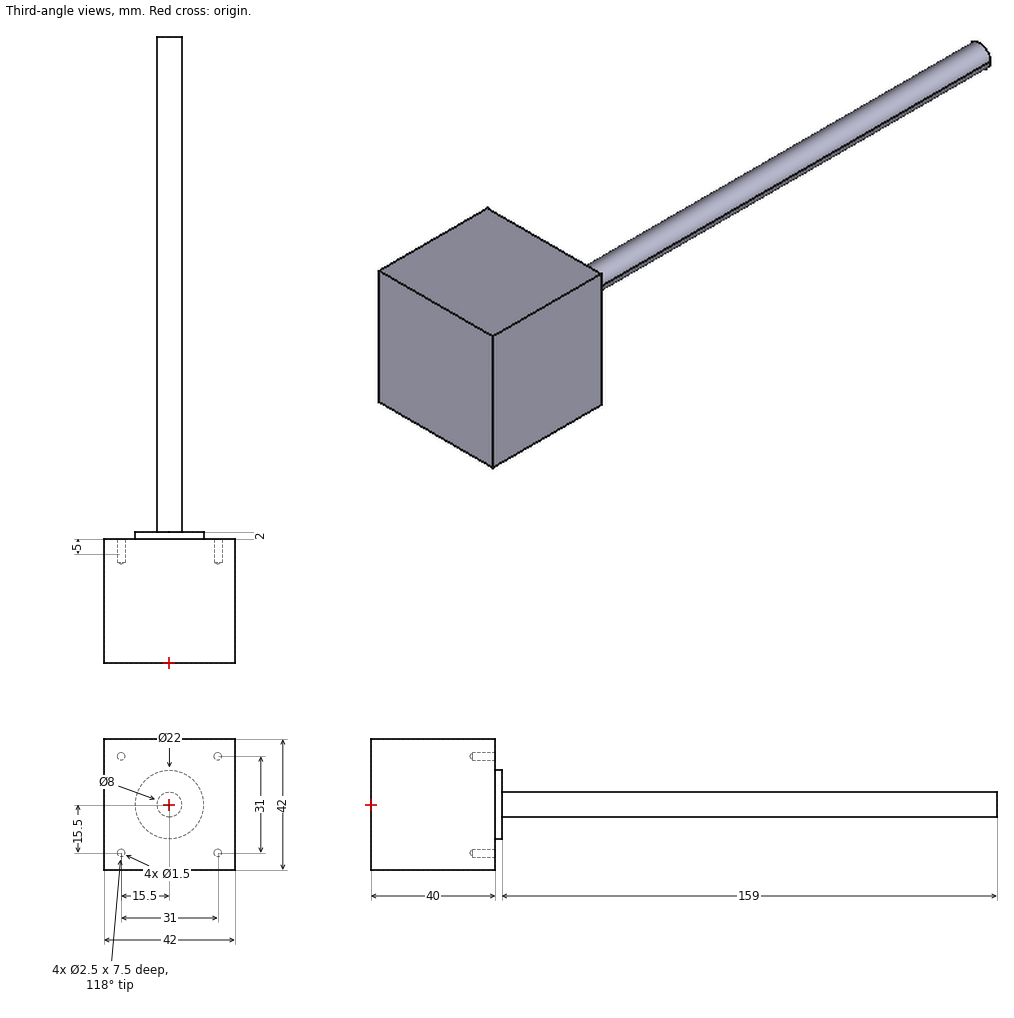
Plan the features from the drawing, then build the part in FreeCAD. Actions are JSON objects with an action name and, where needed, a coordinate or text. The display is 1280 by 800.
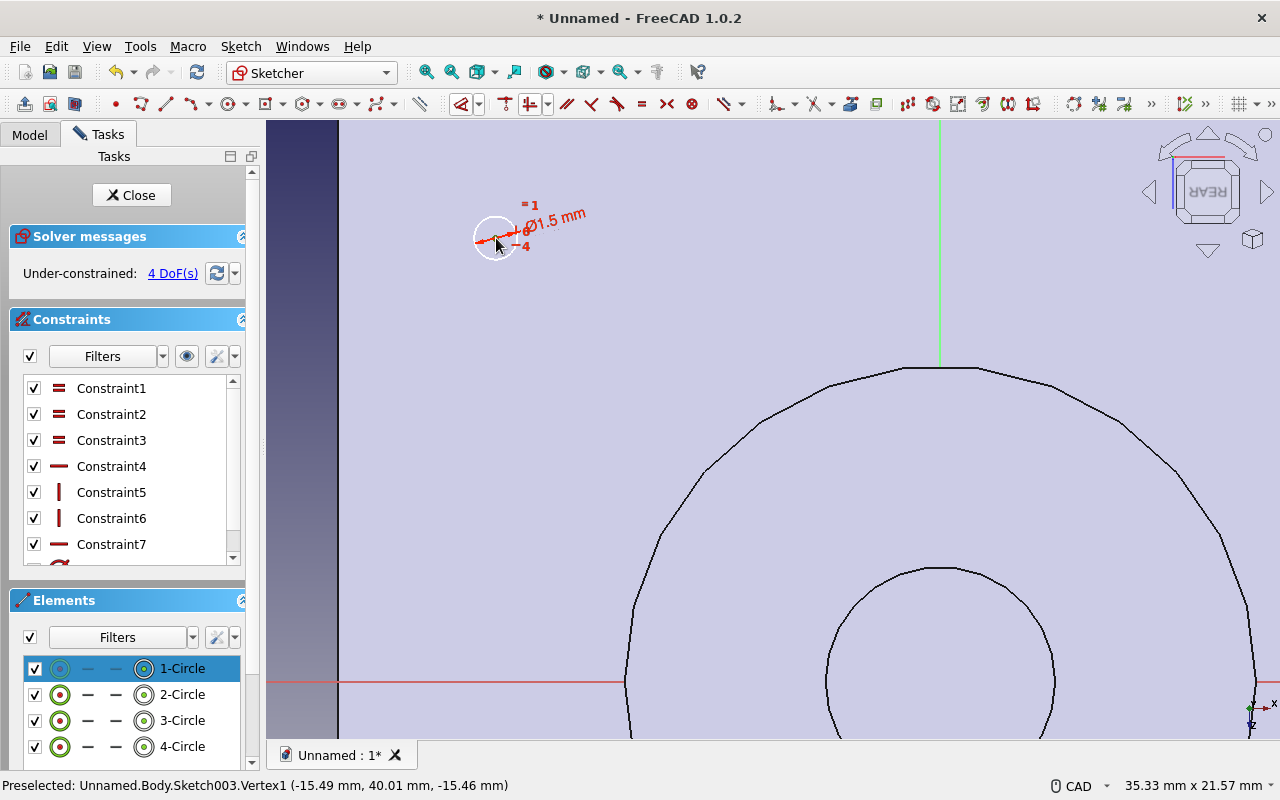
{"action": "scroll", "coordinate": [512, 224], "scroll_direction": "down", "scroll_amount": 4}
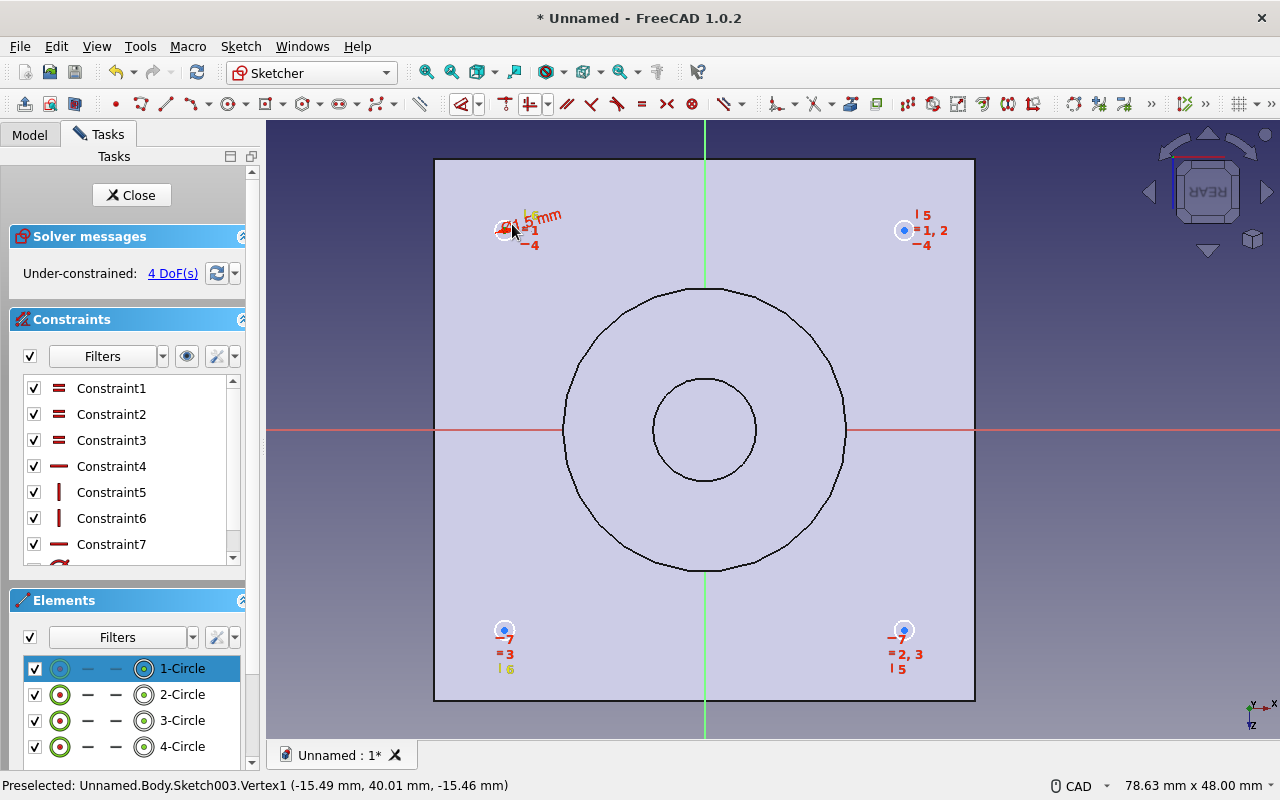
{"action": "left_click", "coordinate": [904, 230]}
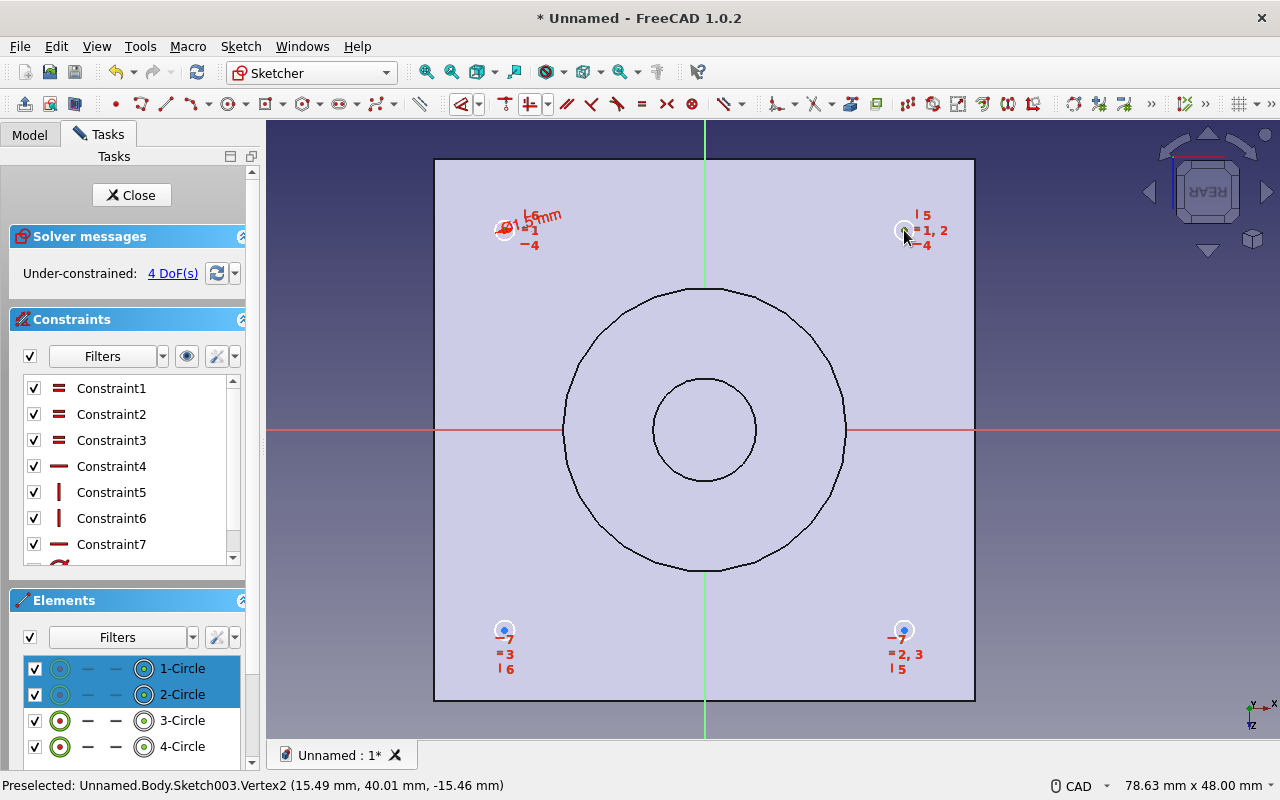
{"action": "key", "text": "l"}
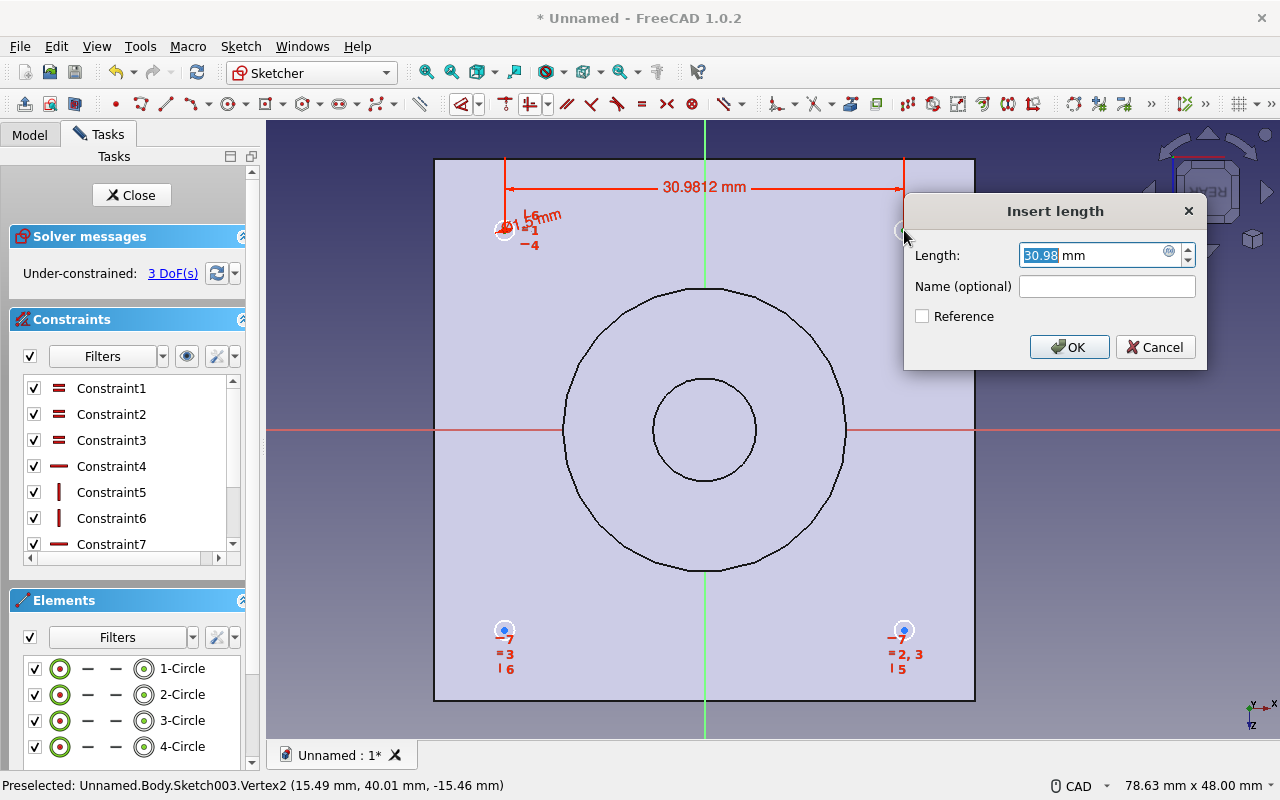
{"action": "type", "text": "31"}
{"action": "key", "text": "Return"}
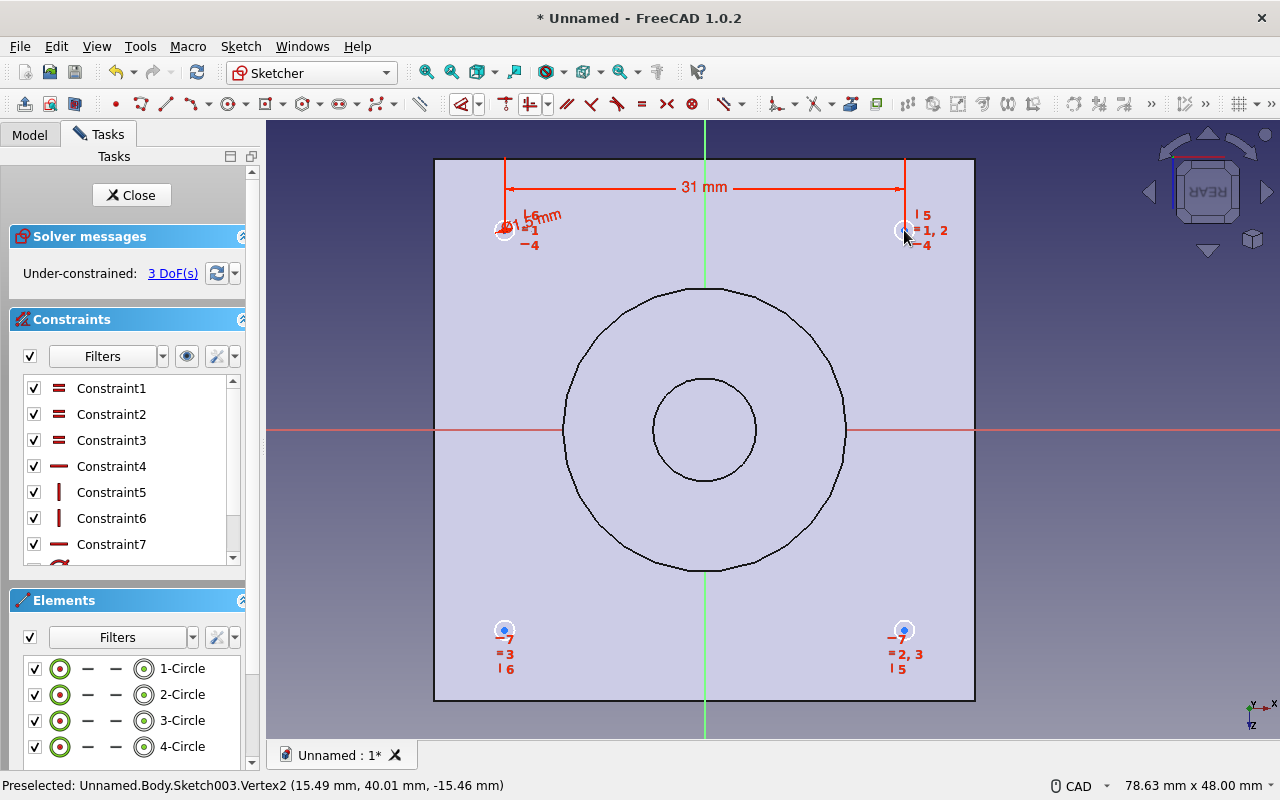
{"action": "left_click", "coordinate": [905, 230]}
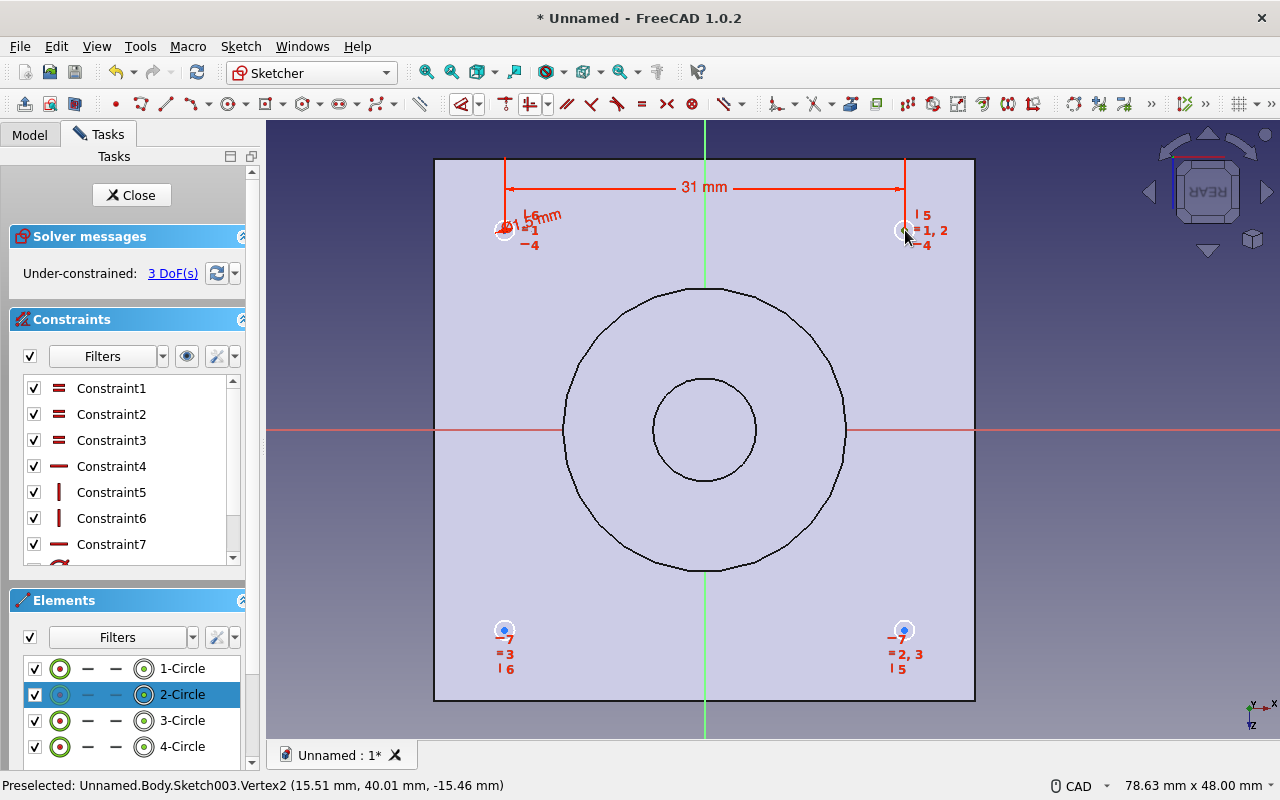
{"action": "left_click", "coordinate": [905, 630]}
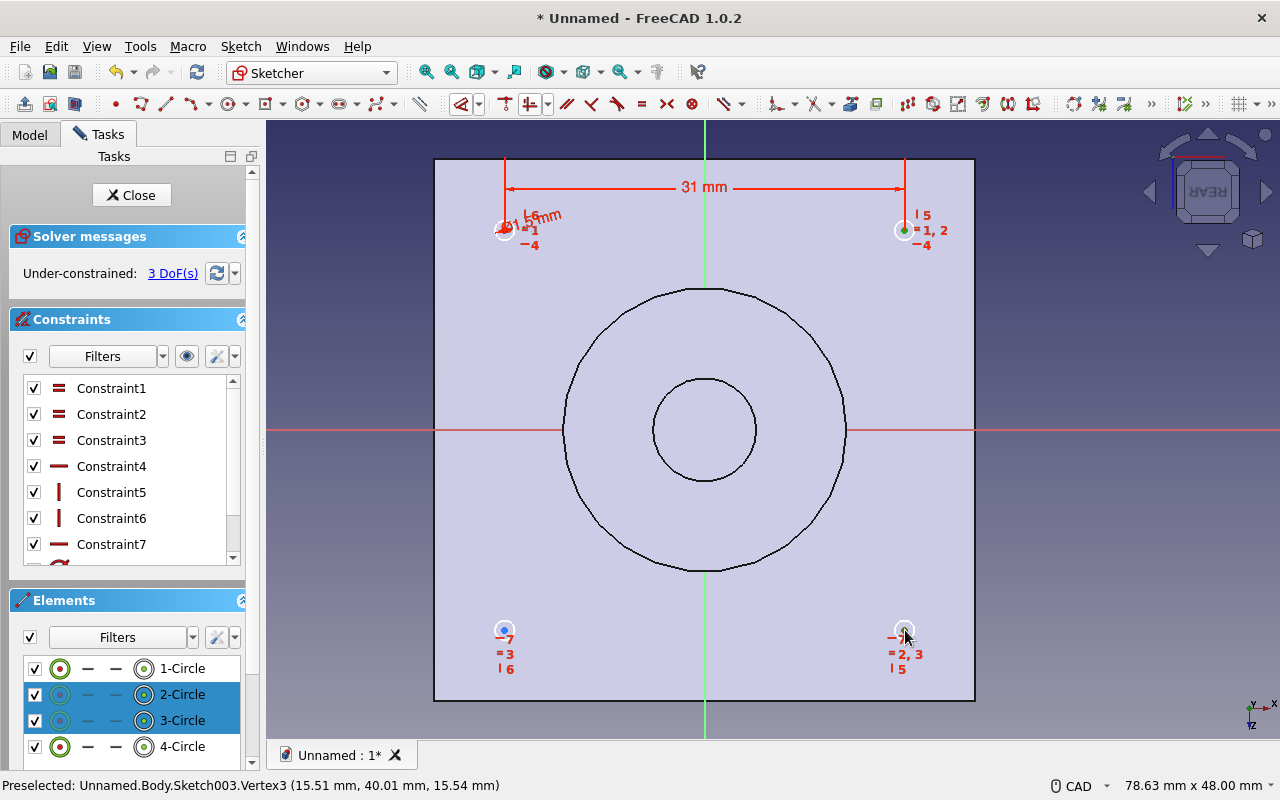
{"action": "key", "text": "i"}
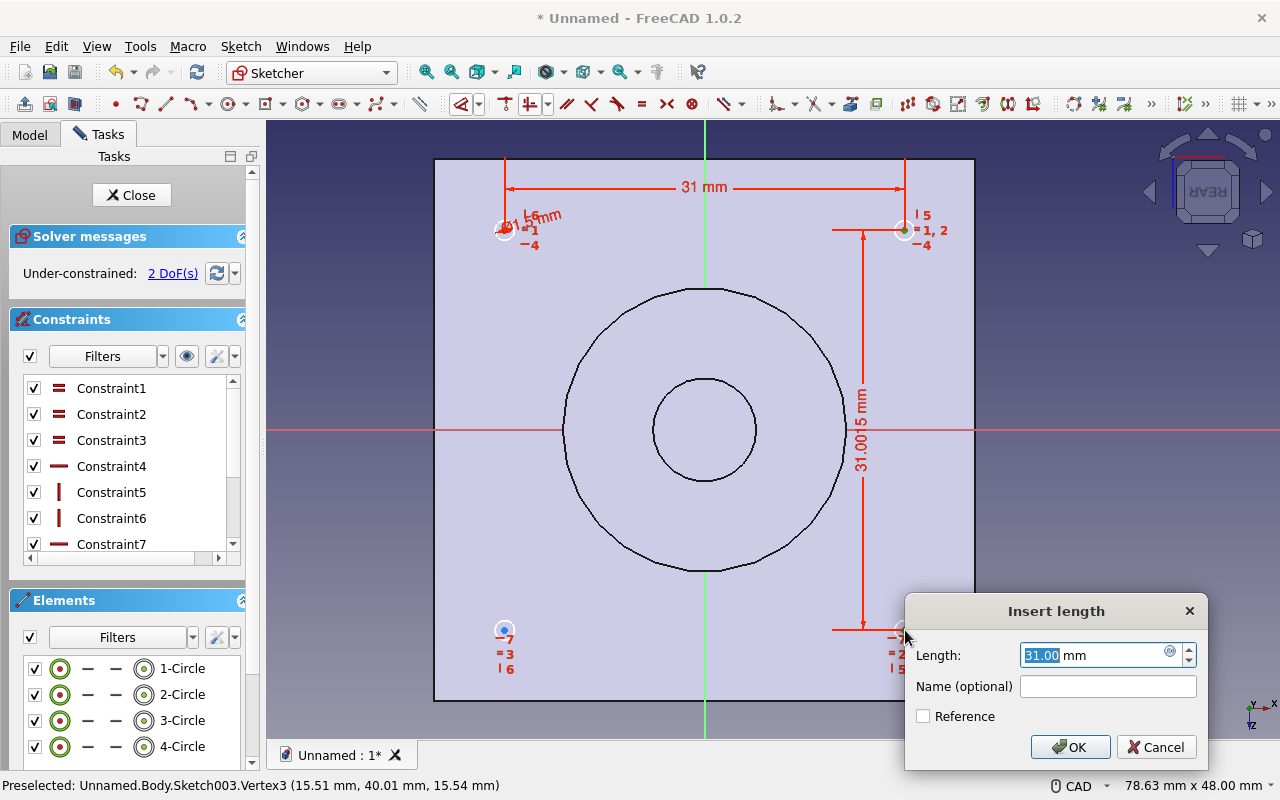
{"action": "type", "text": "31"}
{"action": "key", "text": "Return"}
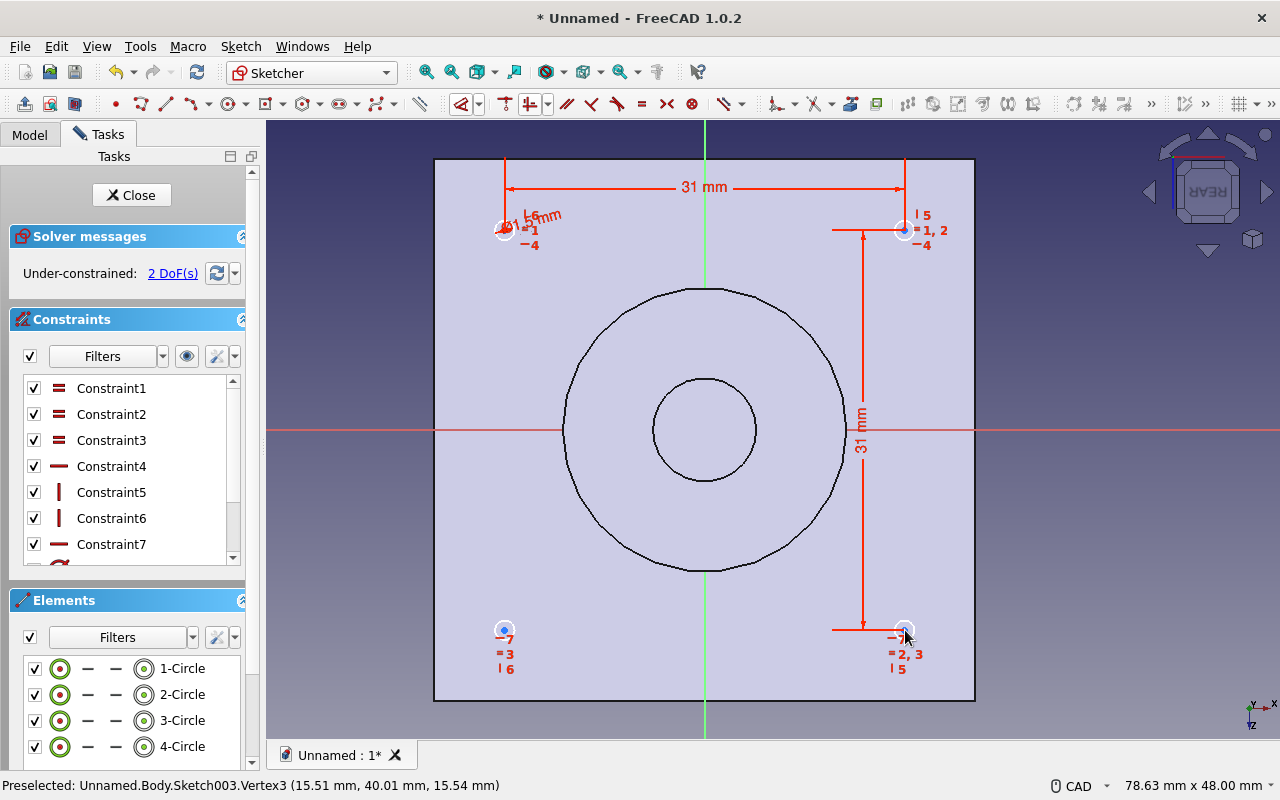
{"action": "left_click", "coordinate": [505, 230]}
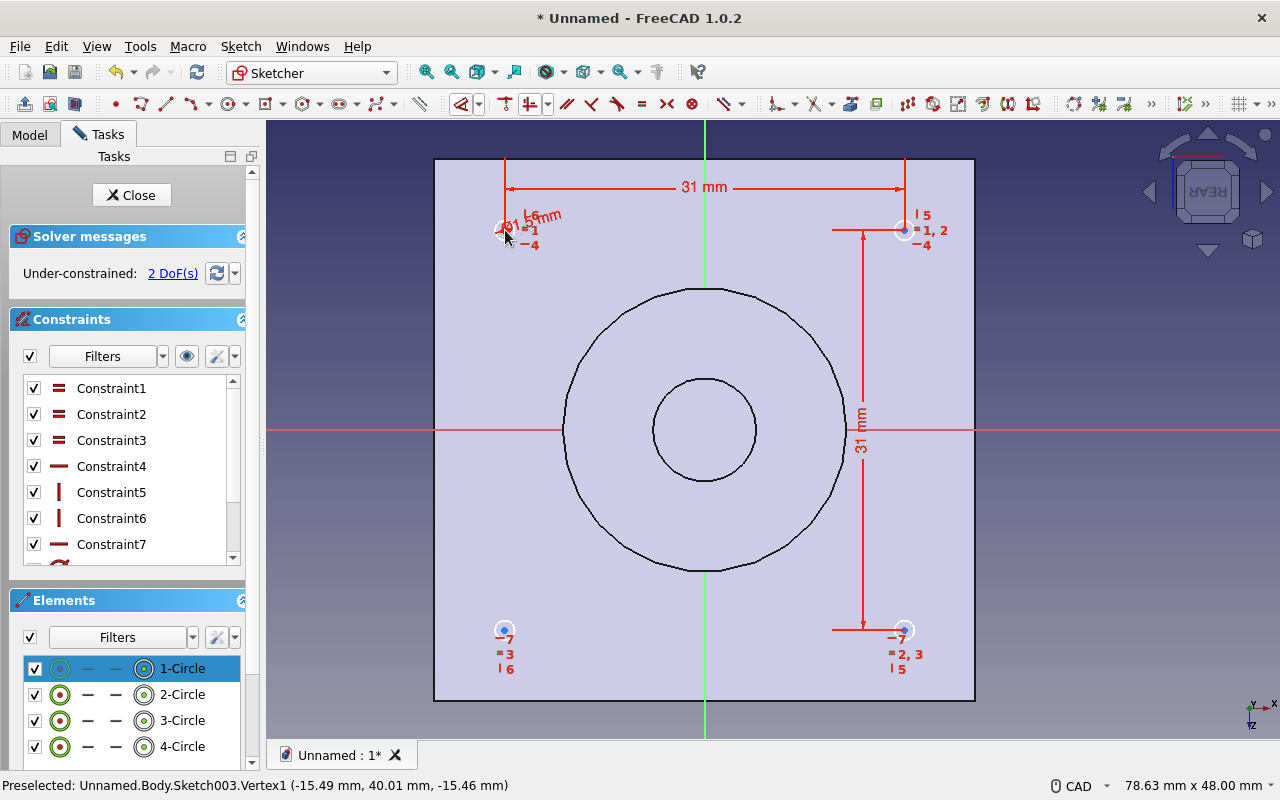
{"action": "key", "text": "l"}